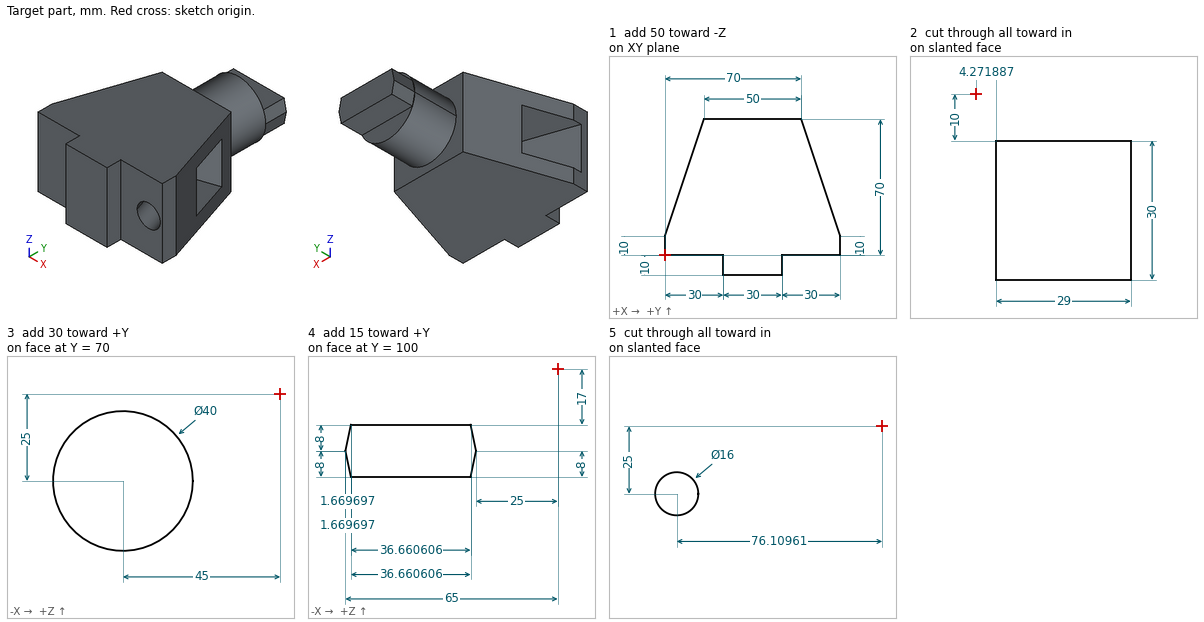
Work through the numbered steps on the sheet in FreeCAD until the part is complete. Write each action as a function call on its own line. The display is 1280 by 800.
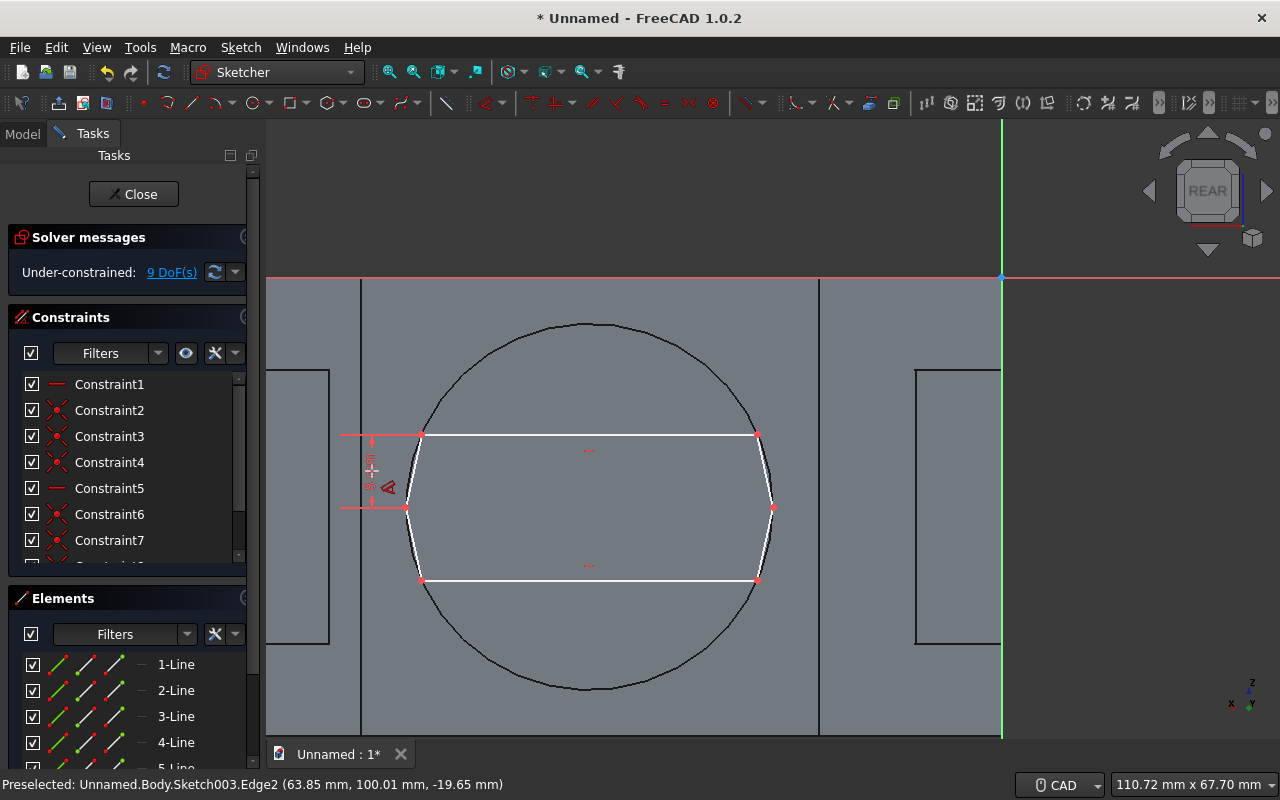
click(411, 530)
click(372, 544)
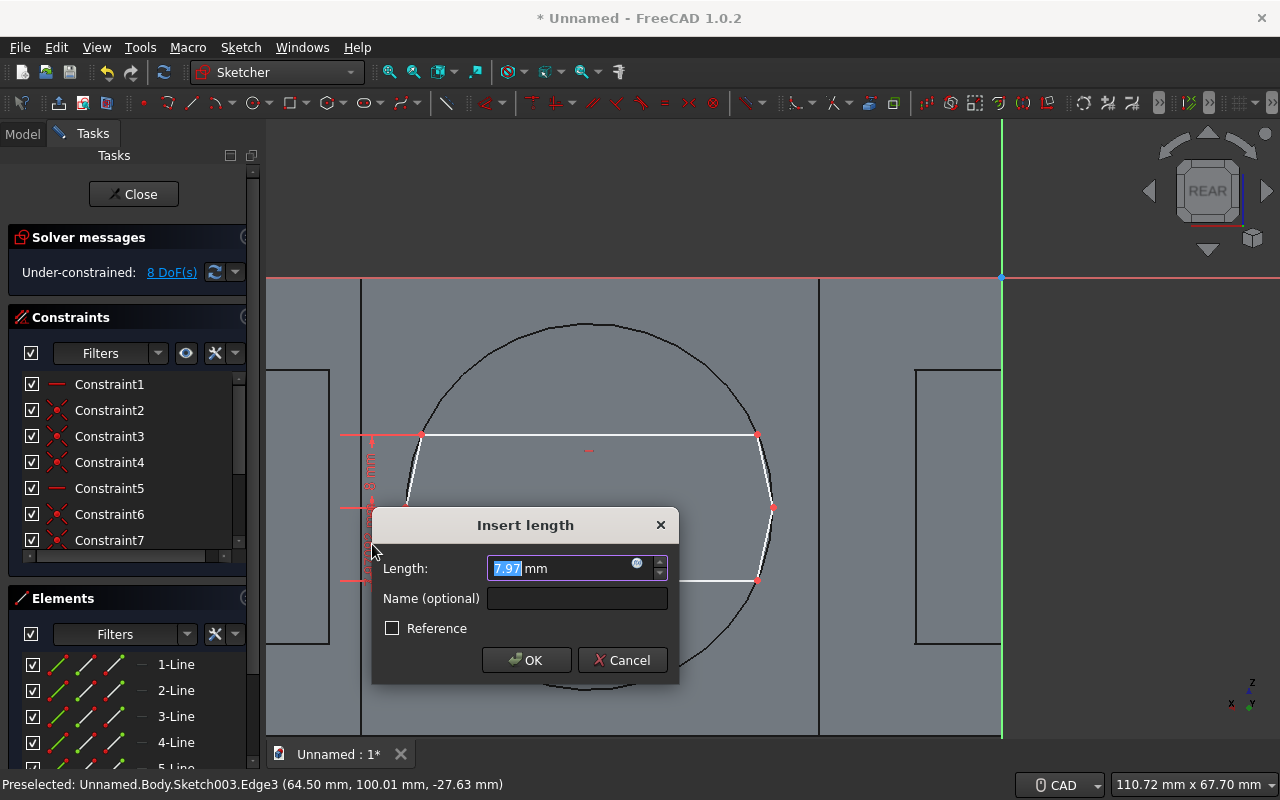
text(8)
key(Return)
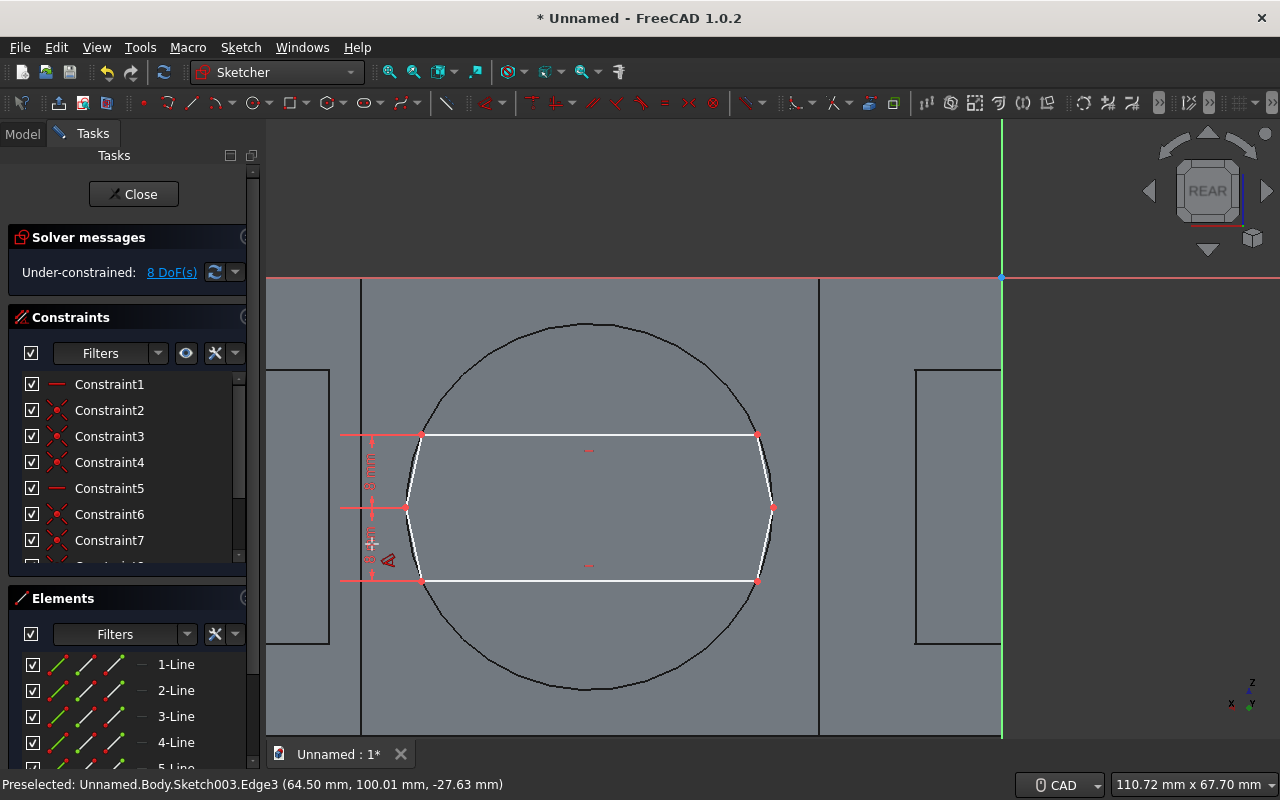
click(762, 559)
click(807, 545)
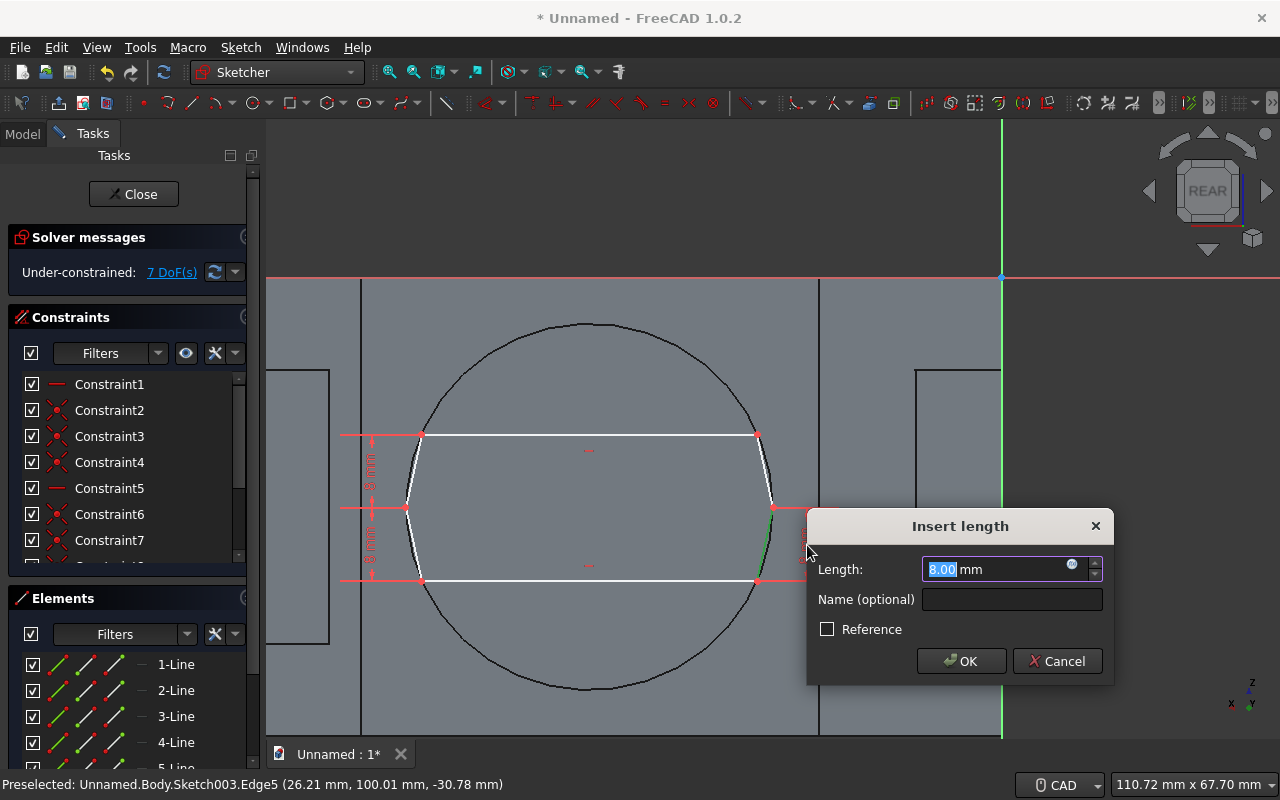
text(8)
key(Return)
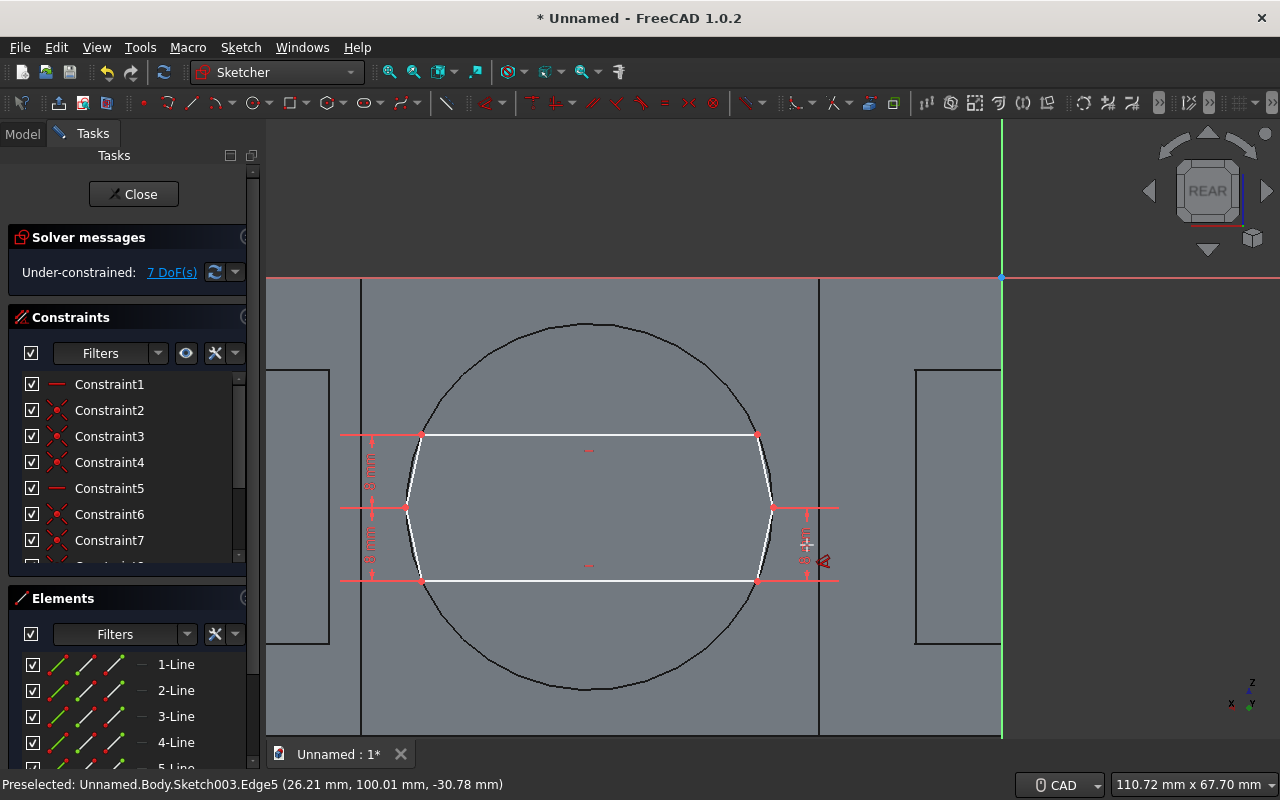
click(757, 435)
click(1036, 356)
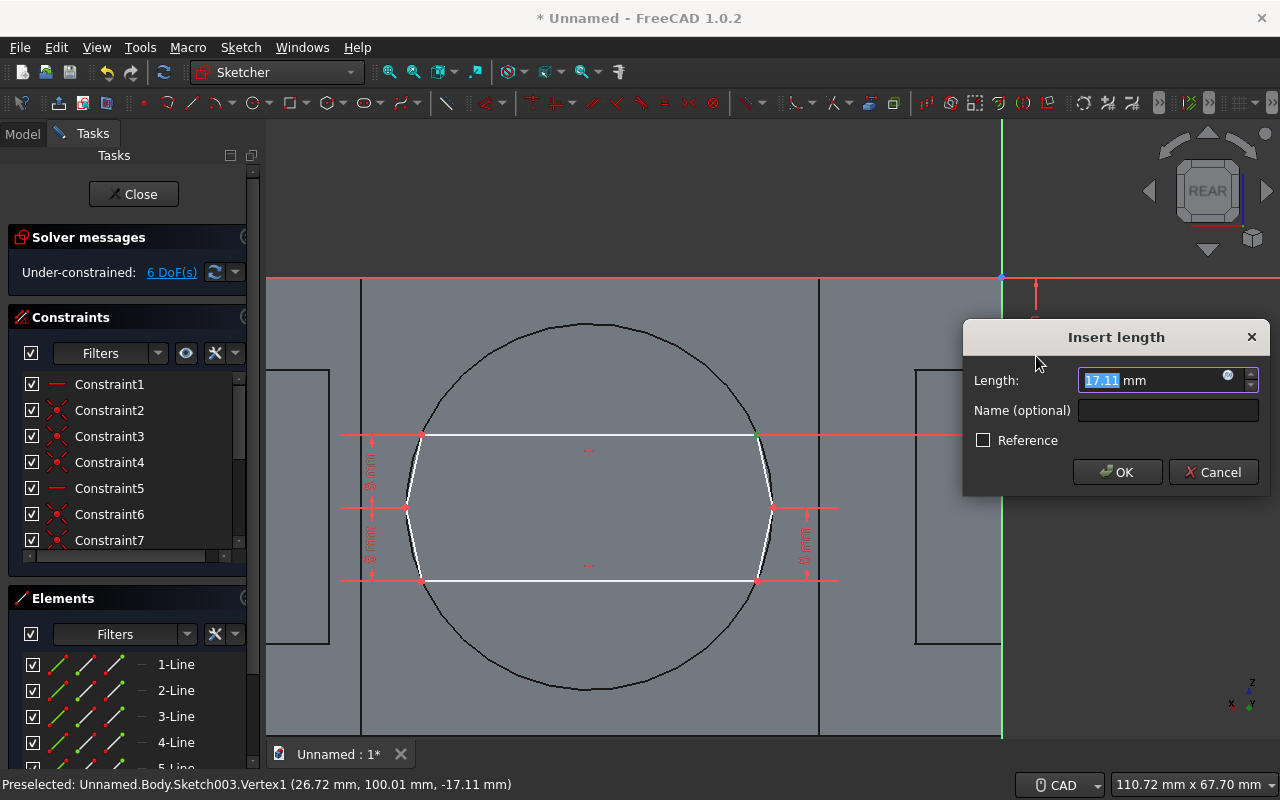
text(17)
key(Return)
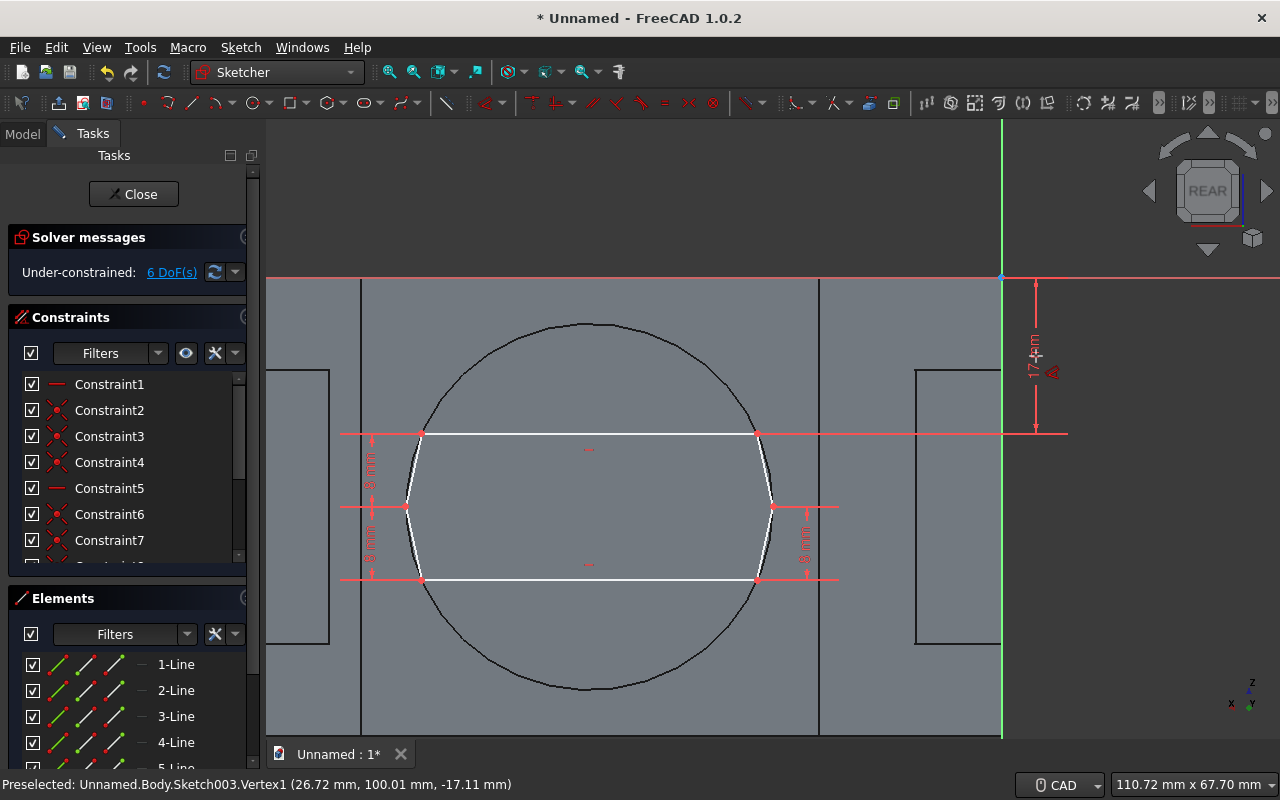
click(406, 507)
click(704, 244)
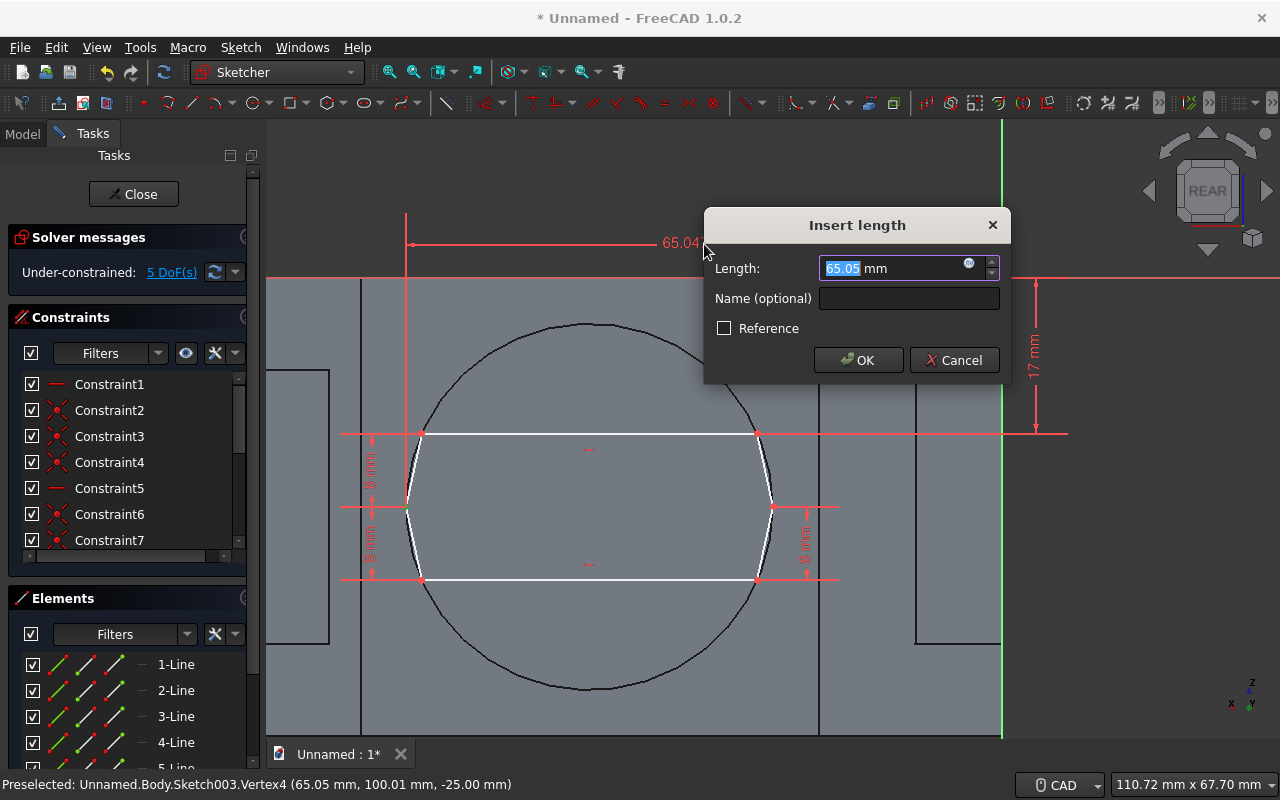
text(65)
key(Return)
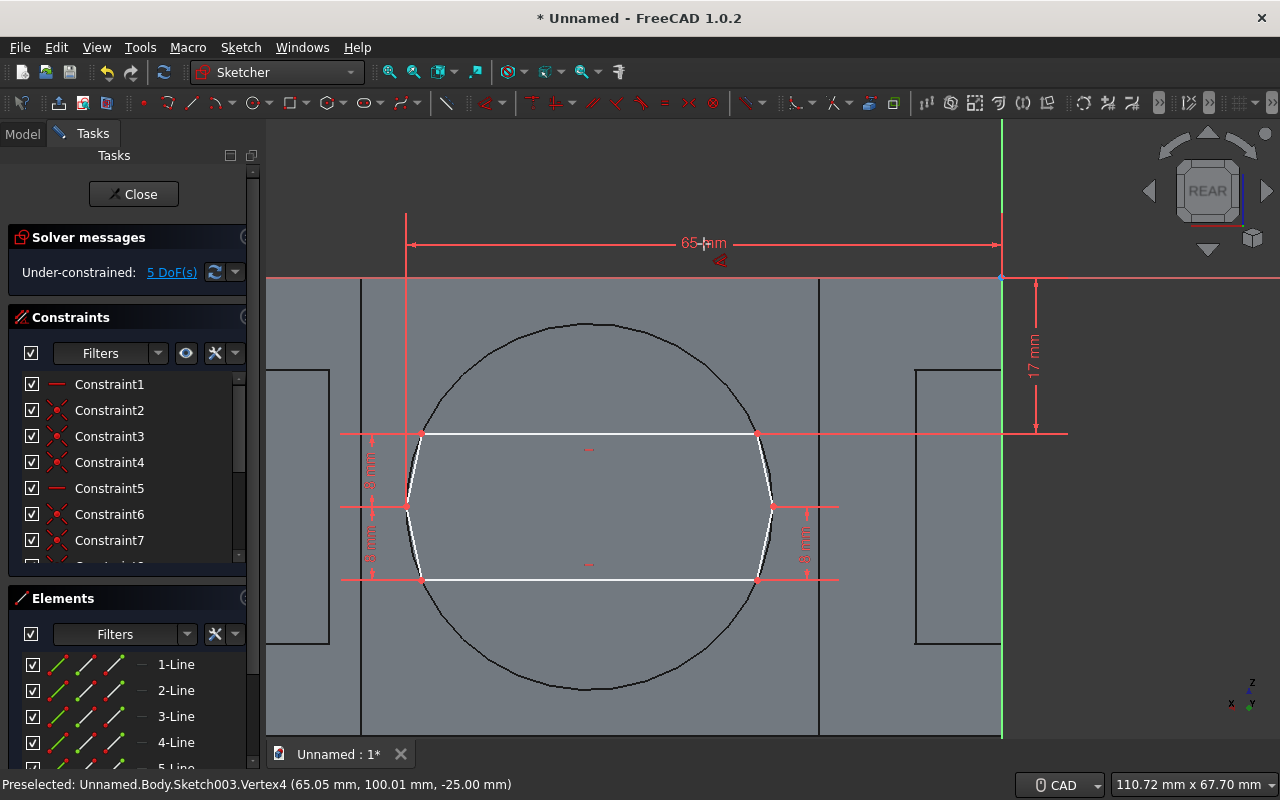
click(773, 507)
click(887, 244)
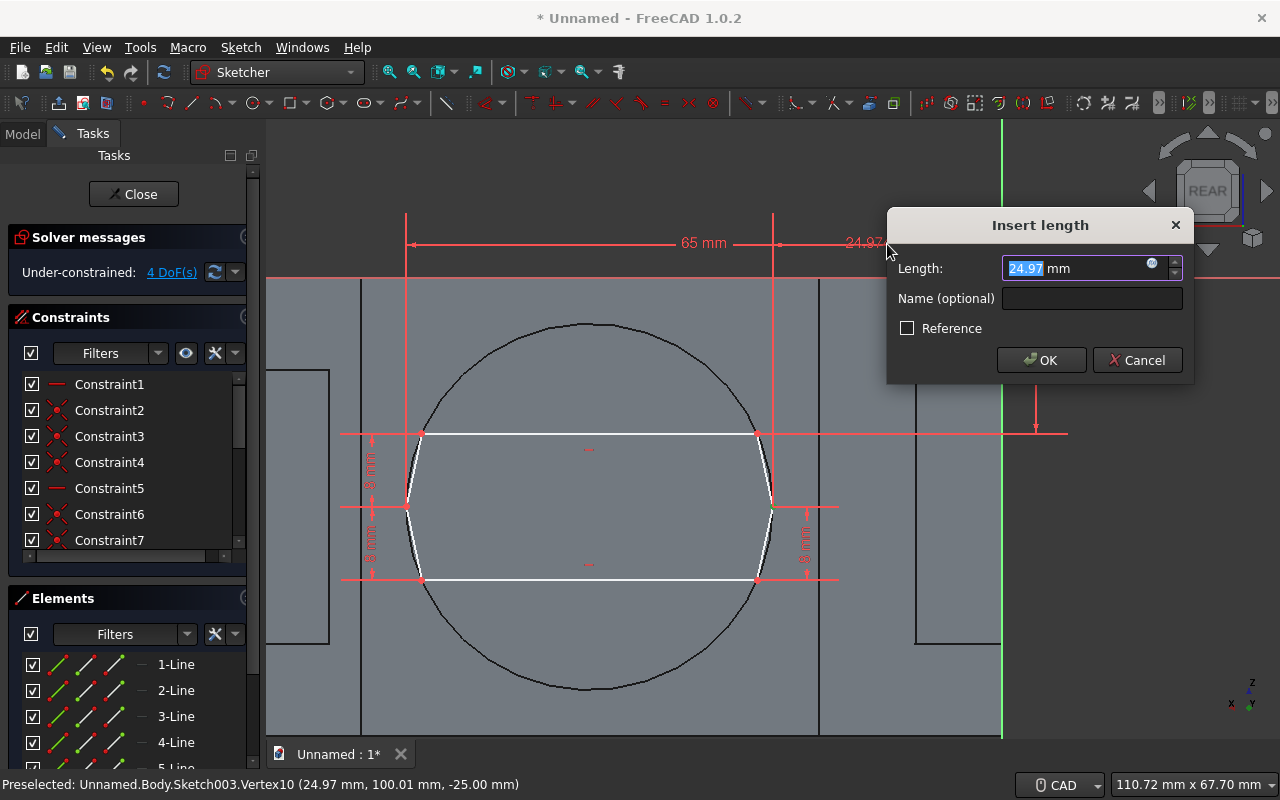
text(25)
key(Return)